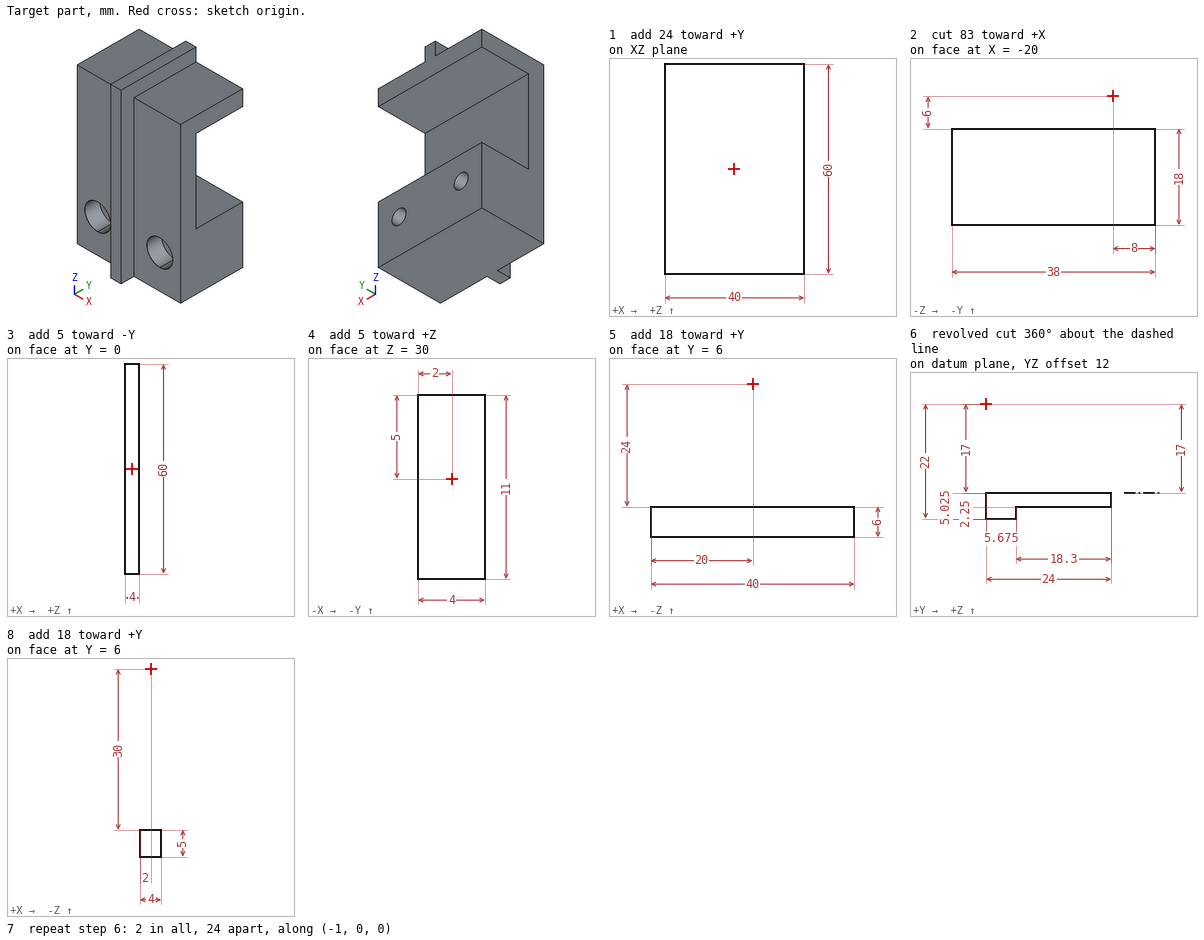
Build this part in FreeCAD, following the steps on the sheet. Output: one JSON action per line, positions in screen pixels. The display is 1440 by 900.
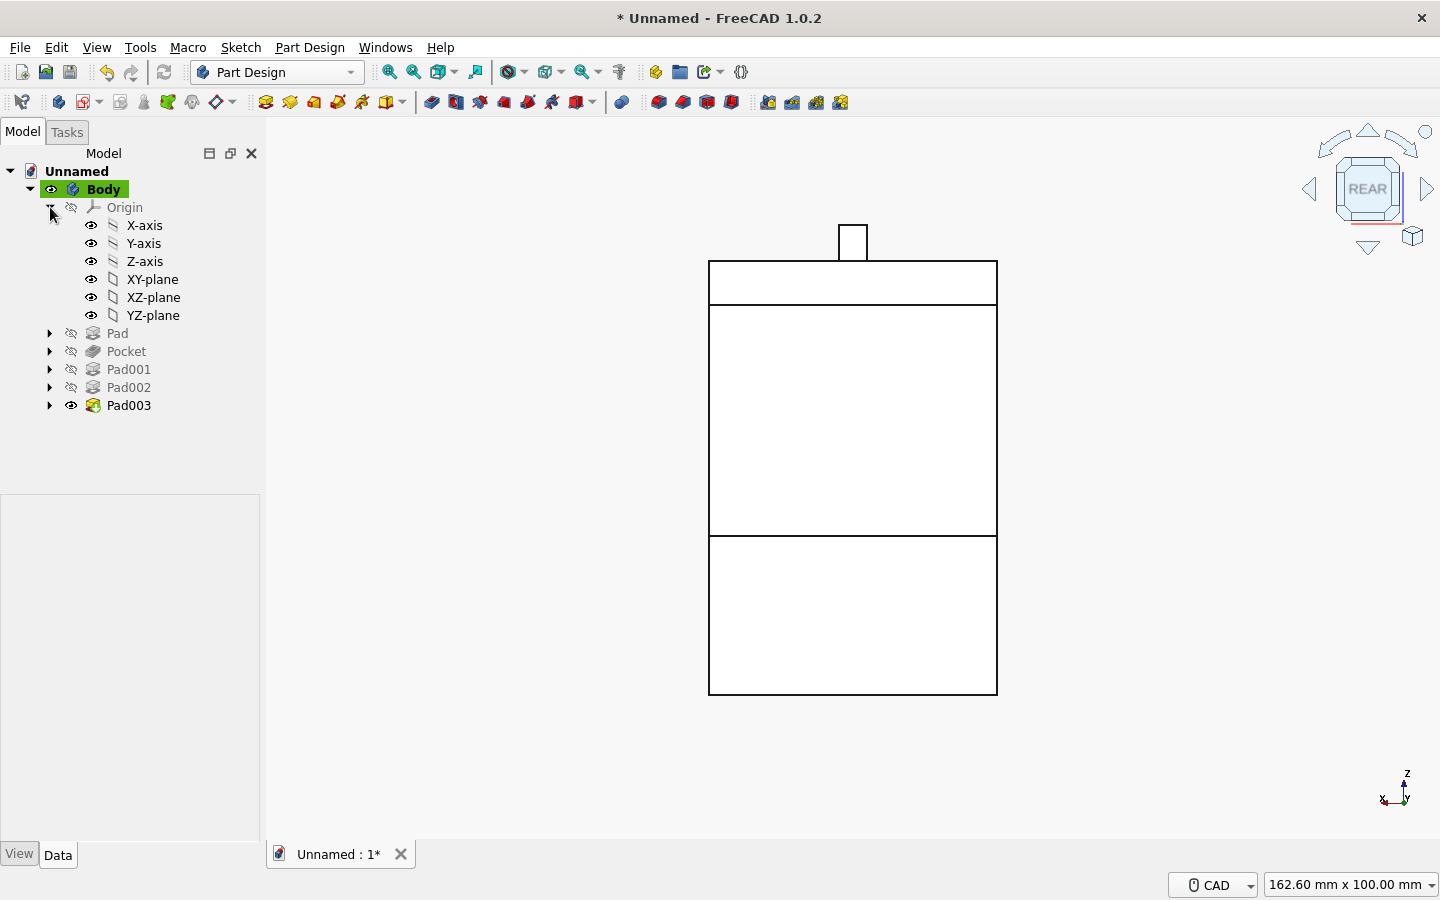
{"action": "left_click", "coordinate": [136, 315]}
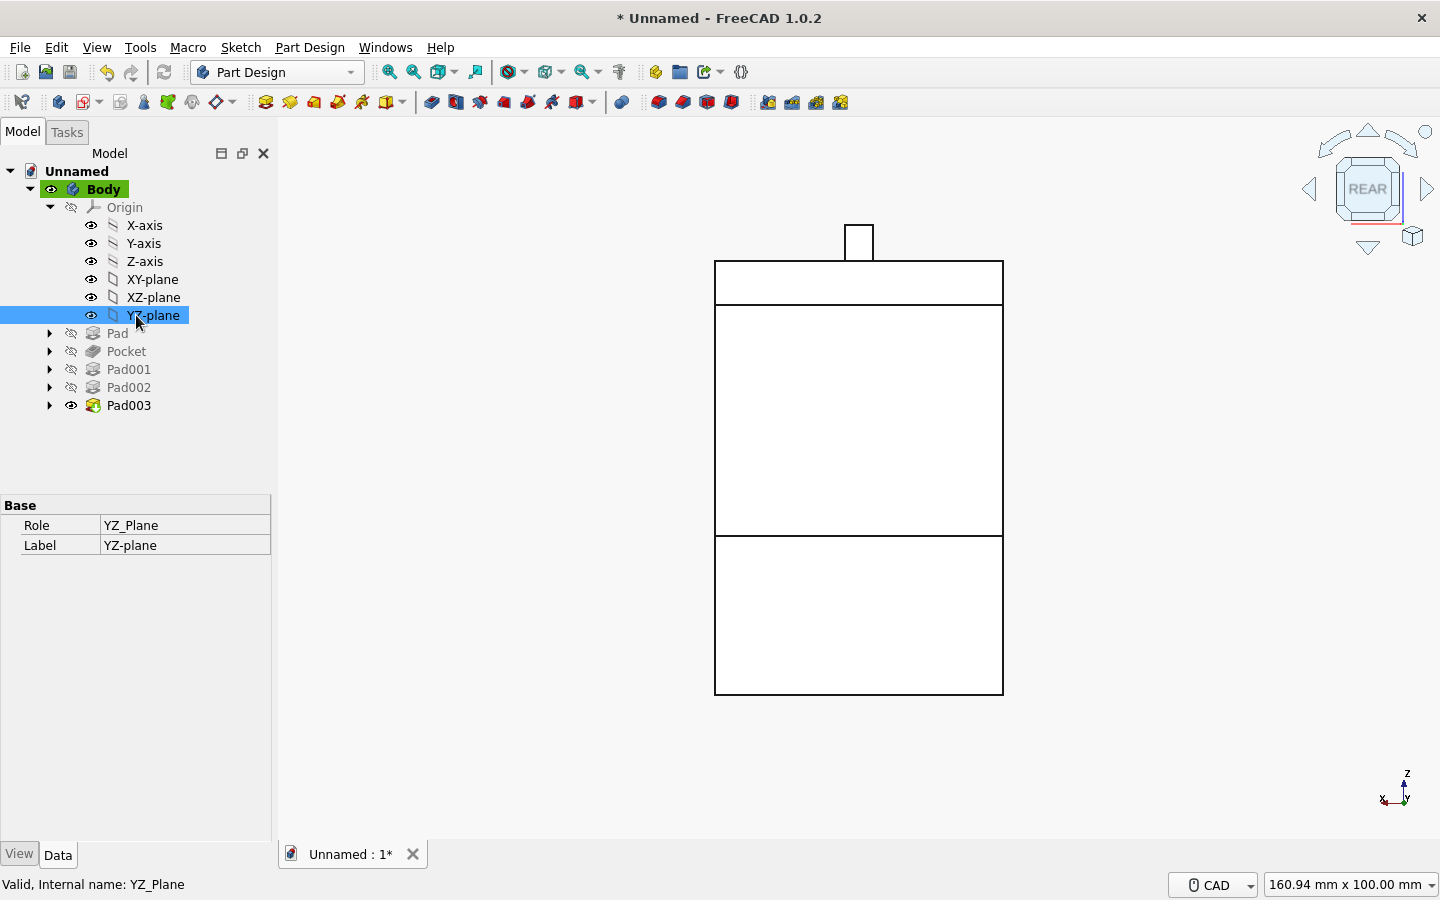
{"action": "left_click", "coordinate": [216, 102]}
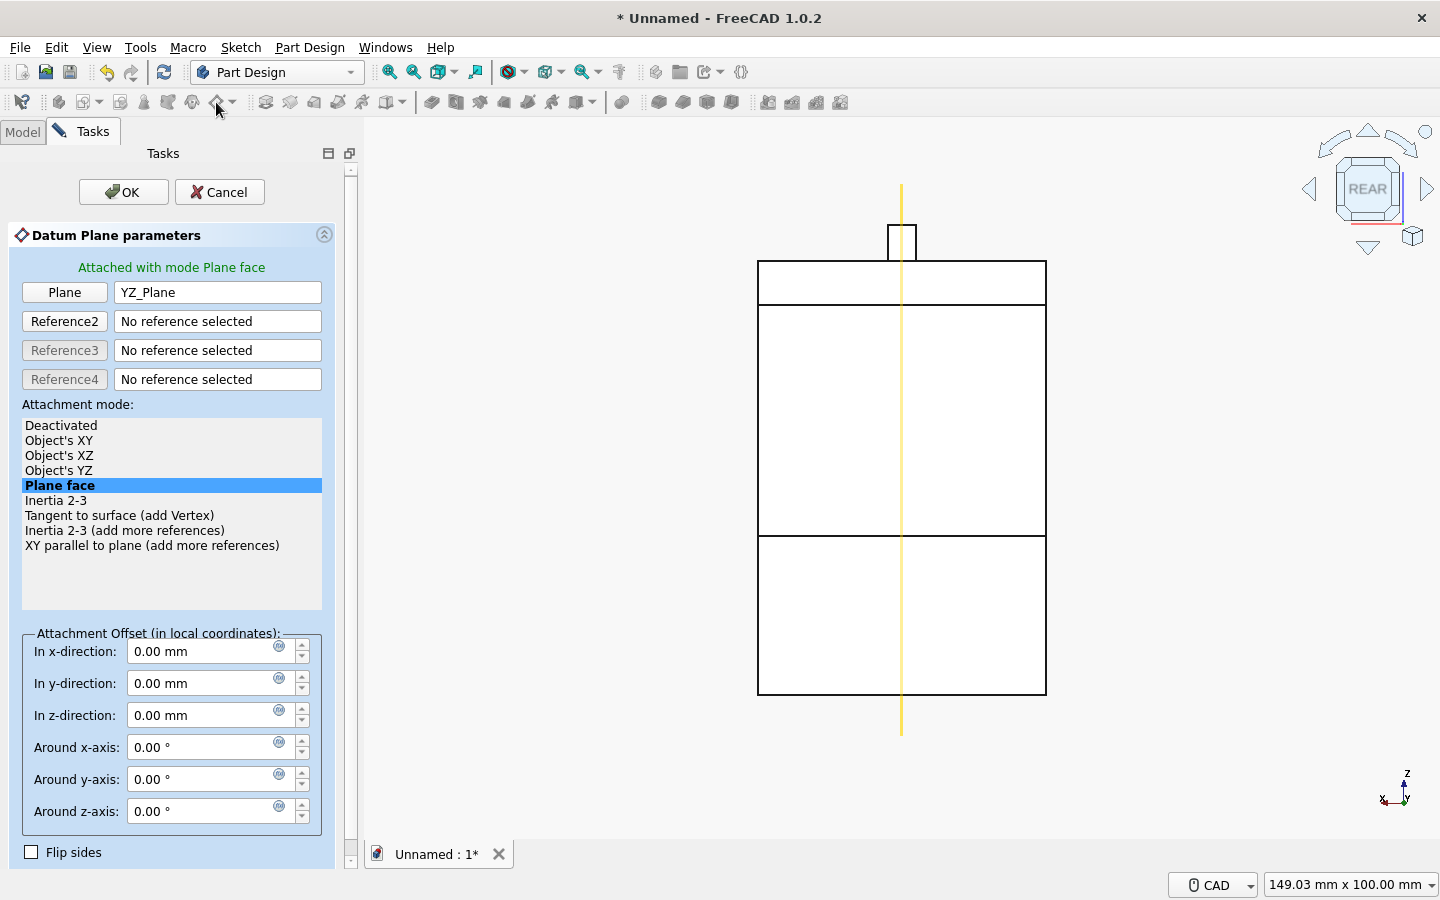
{"action": "triple_click", "coordinate": [210, 715]}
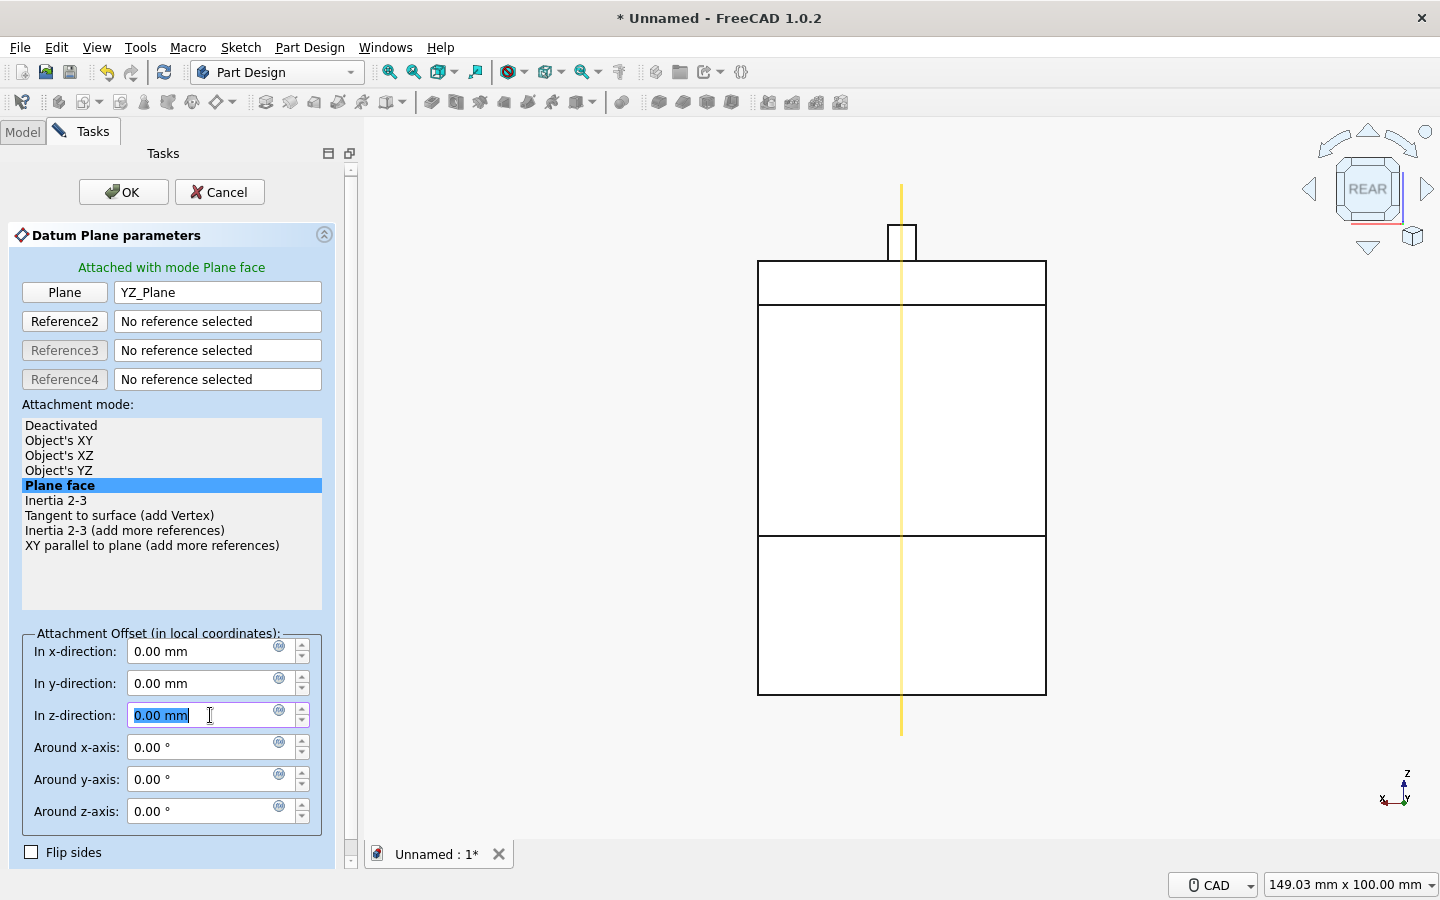
{"action": "type", "text": "12"}
{"action": "key", "text": "Tab"}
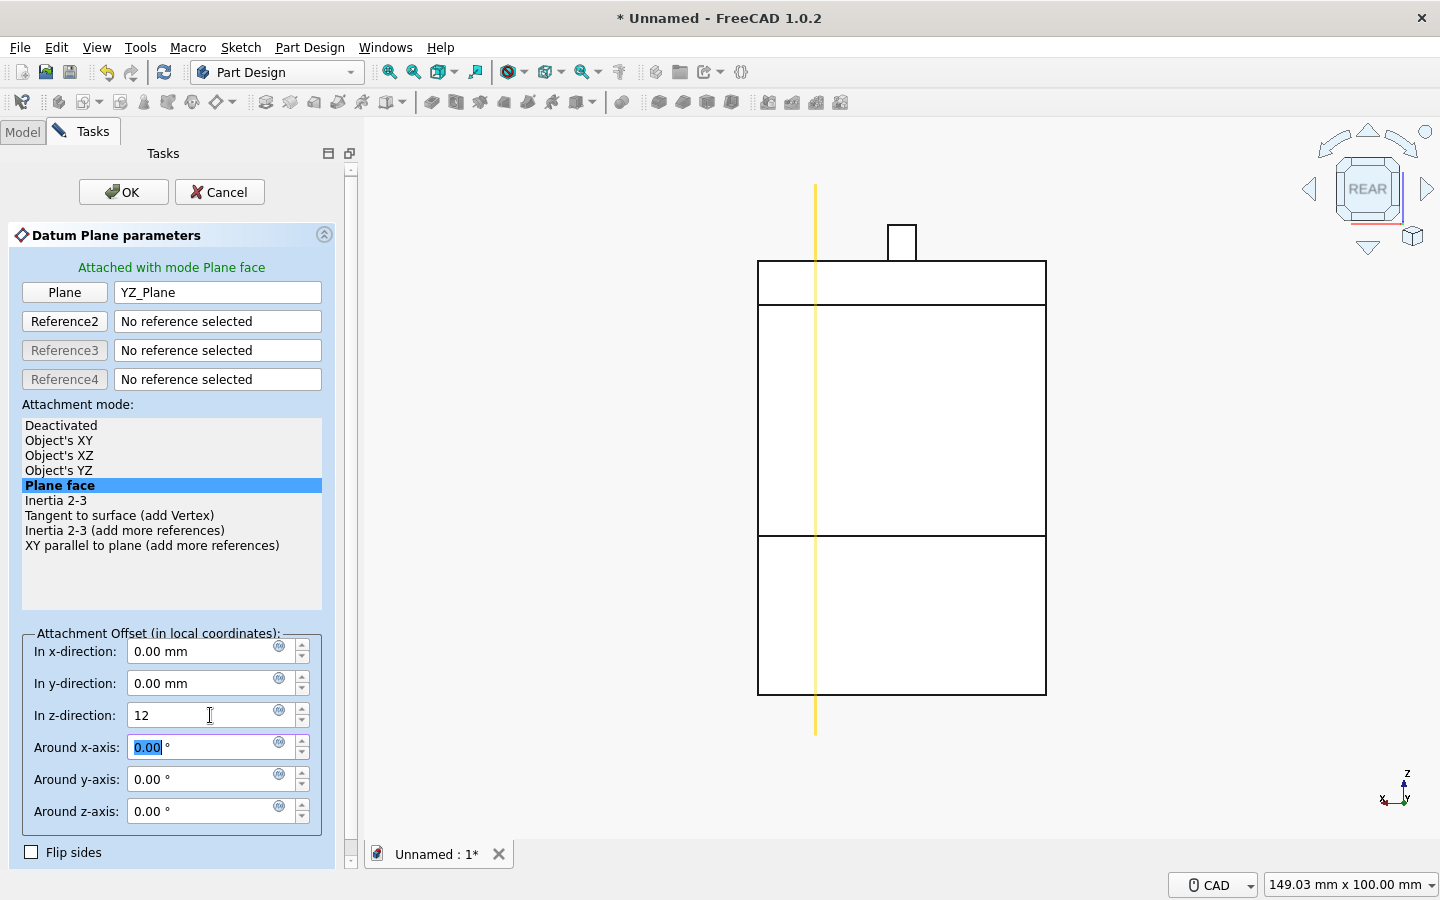
{"action": "left_click", "coordinate": [124, 192]}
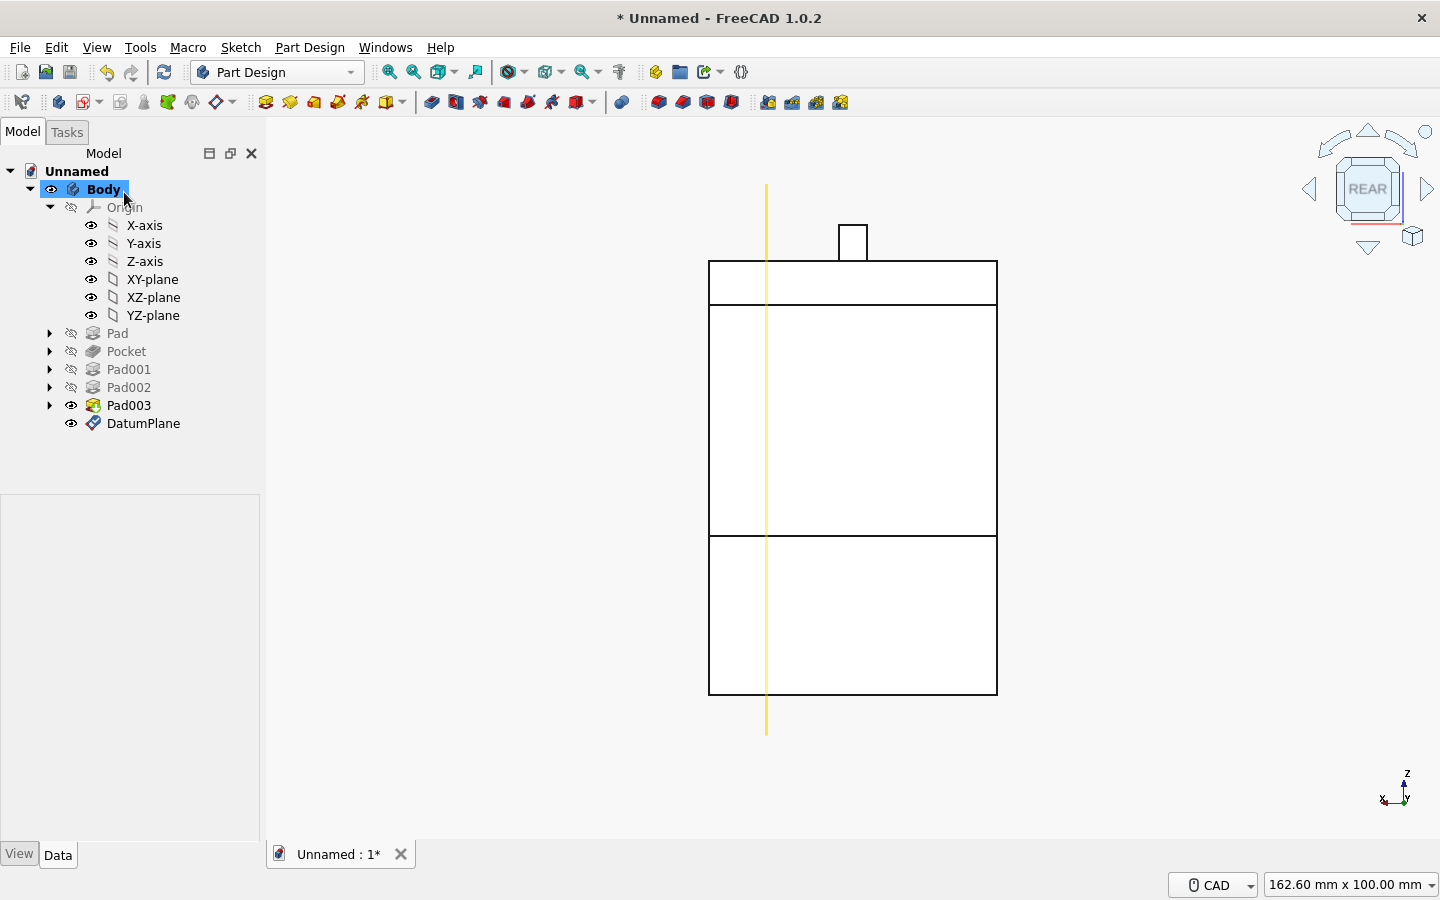
{"action": "left_click", "coordinate": [116, 423]}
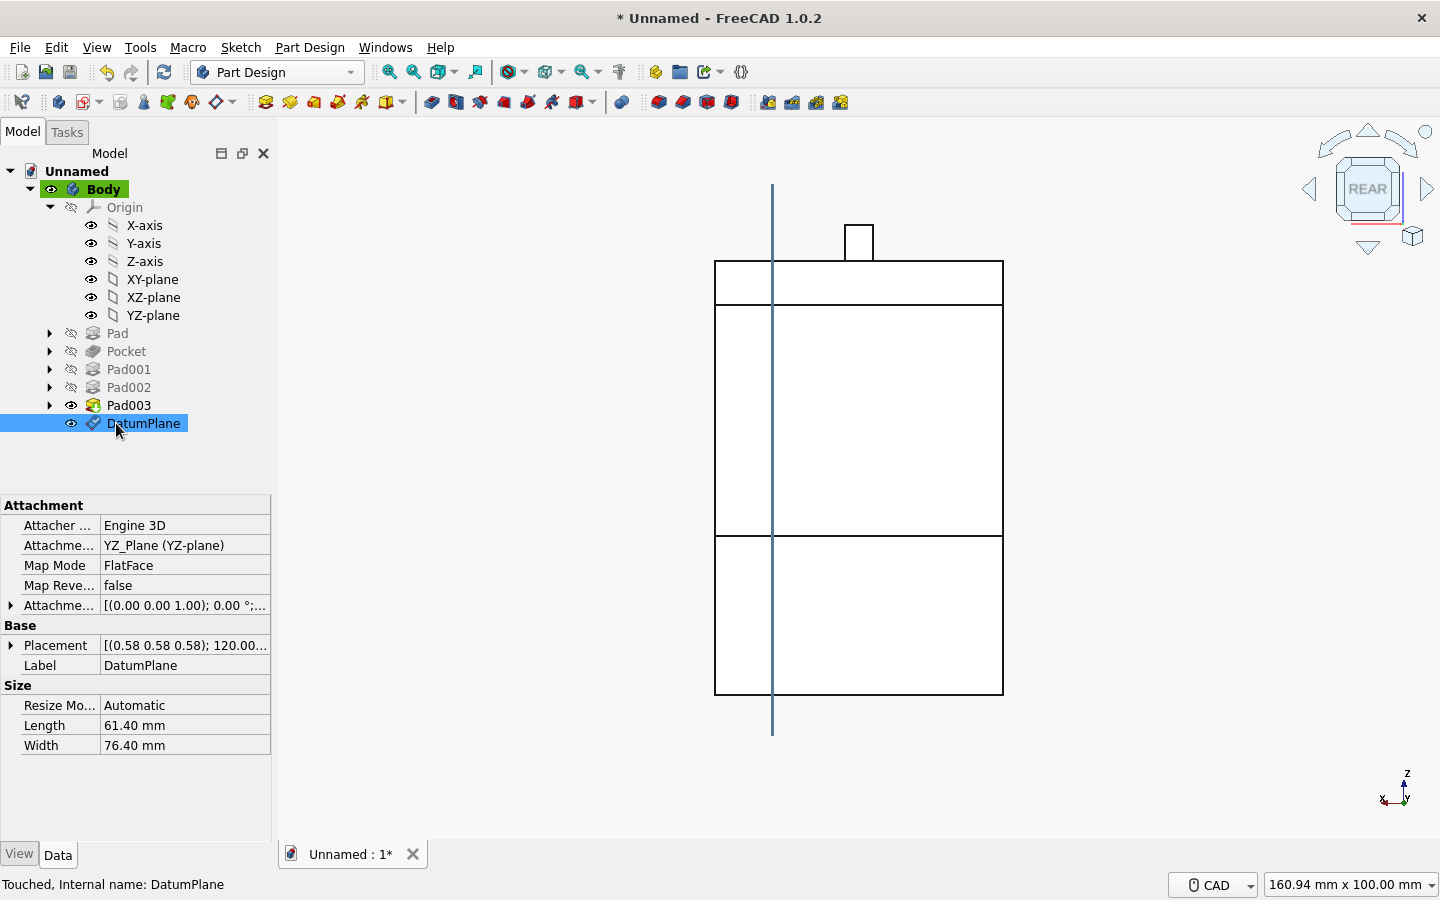
{"action": "left_click", "coordinate": [84, 102]}